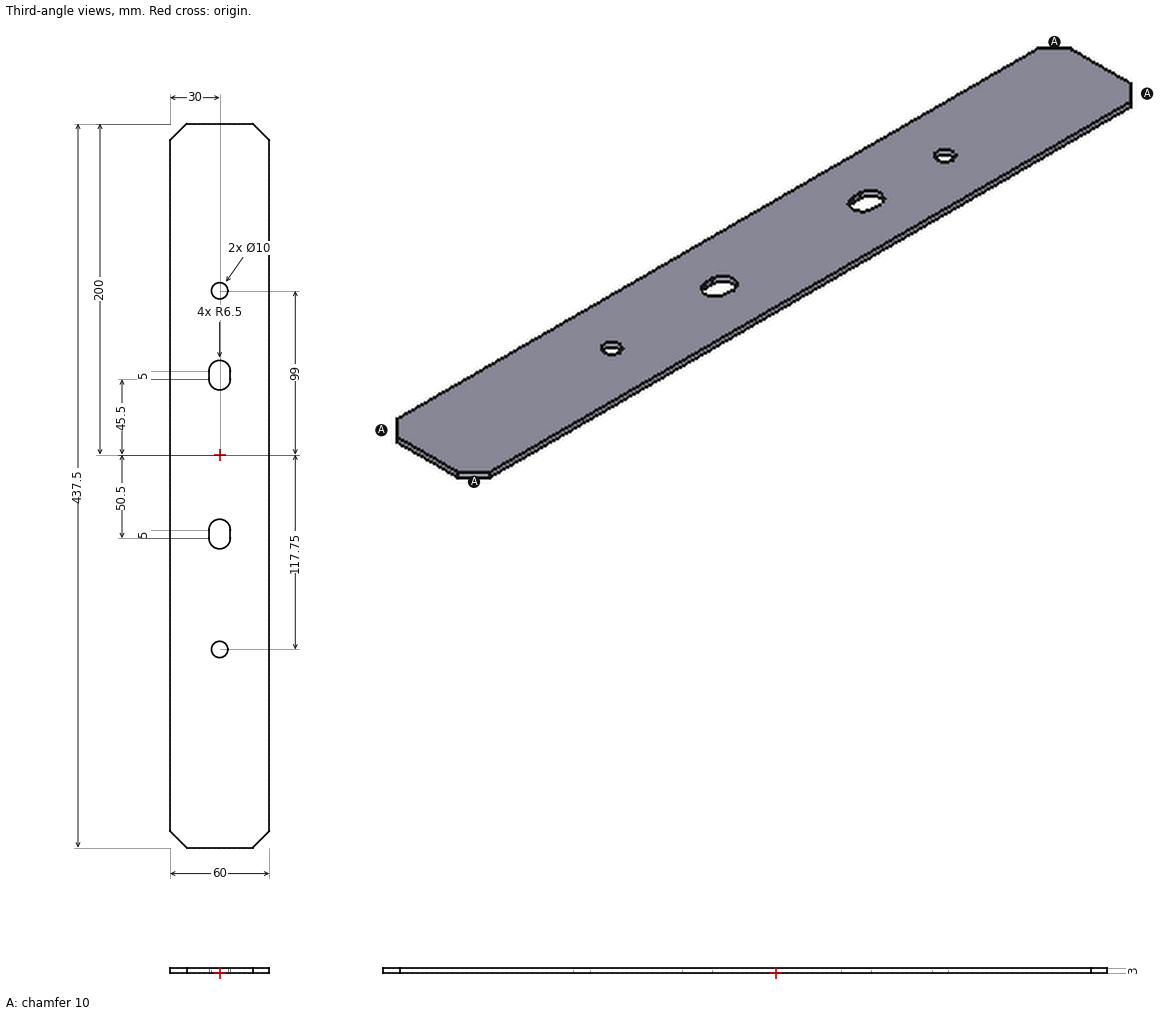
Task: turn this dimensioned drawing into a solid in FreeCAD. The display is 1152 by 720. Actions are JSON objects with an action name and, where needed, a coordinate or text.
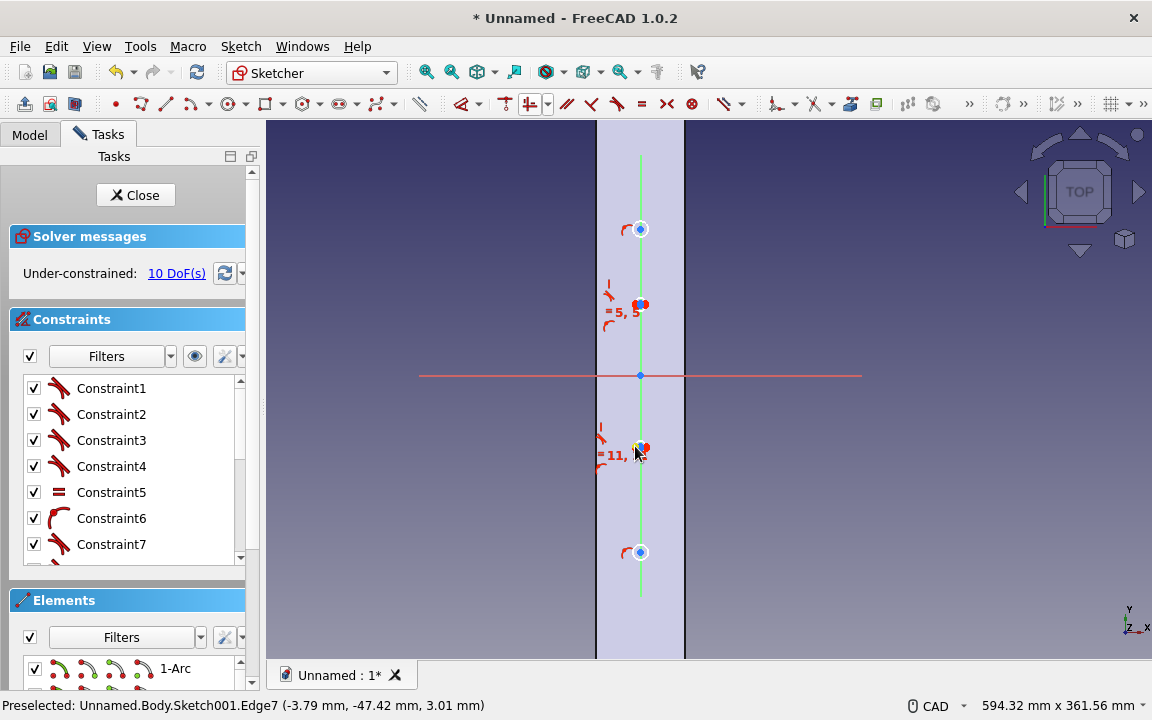
{"action": "scroll", "coordinate": [637, 310], "scroll_direction": "up", "scroll_amount": 8}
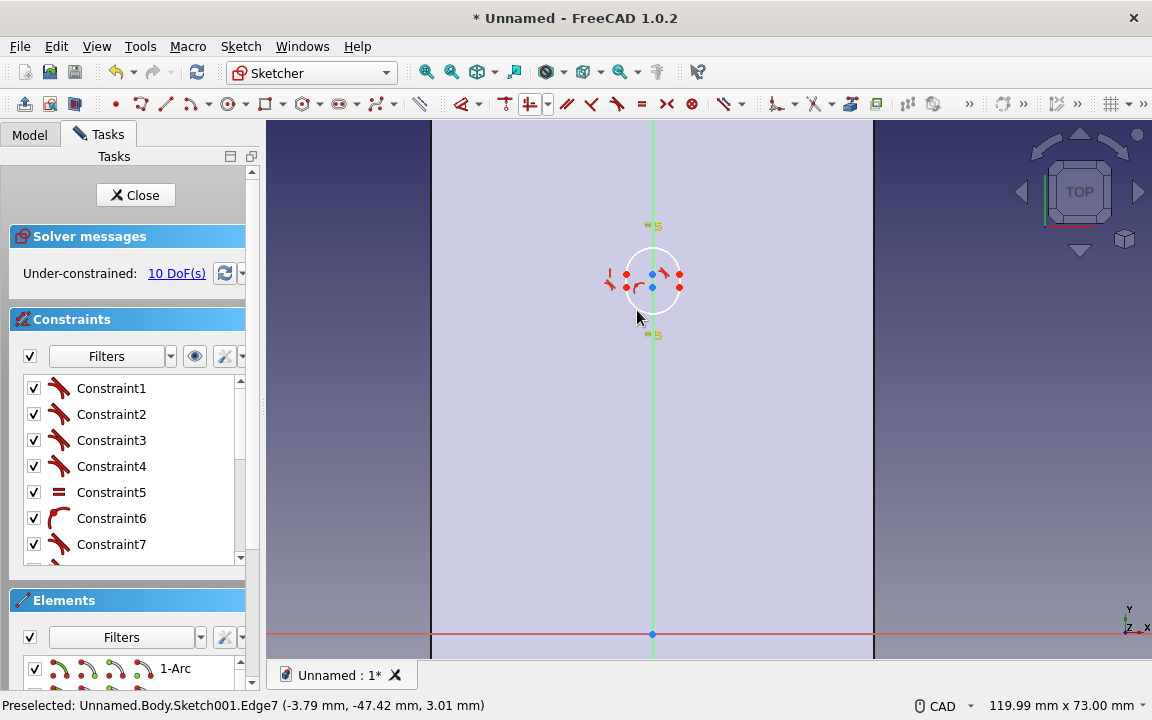
{"action": "left_click", "coordinate": [637, 309]}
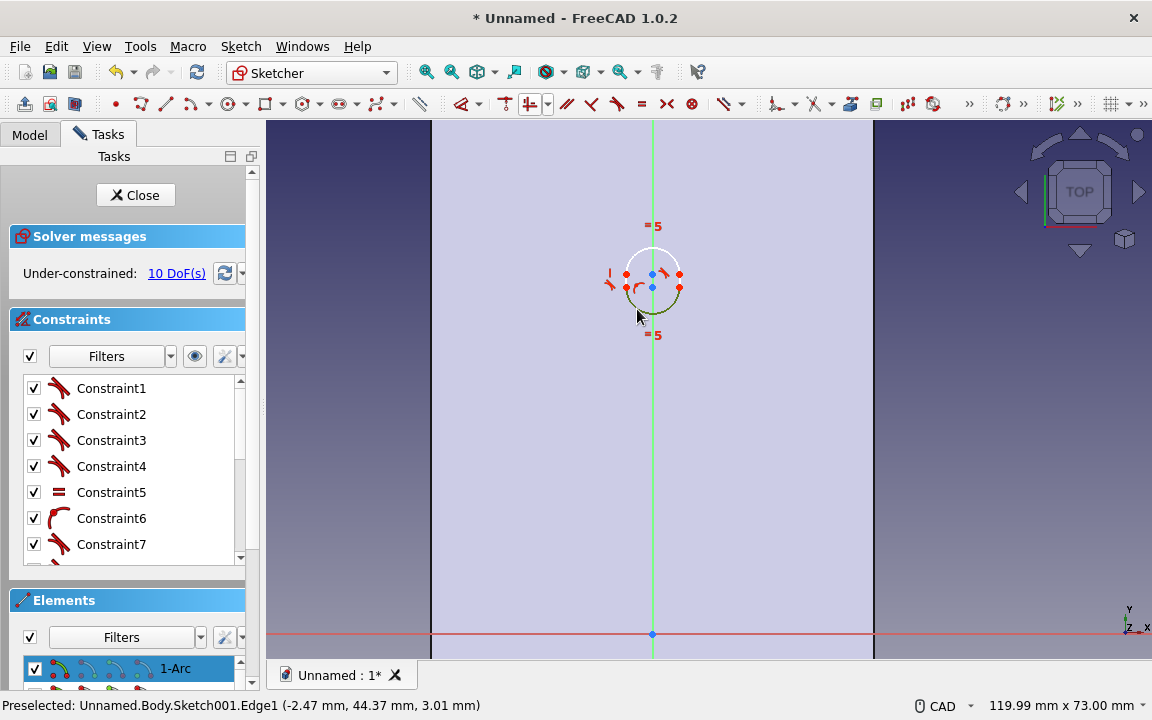
{"action": "scroll", "coordinate": [637, 310], "scroll_direction": "down", "scroll_amount": 8}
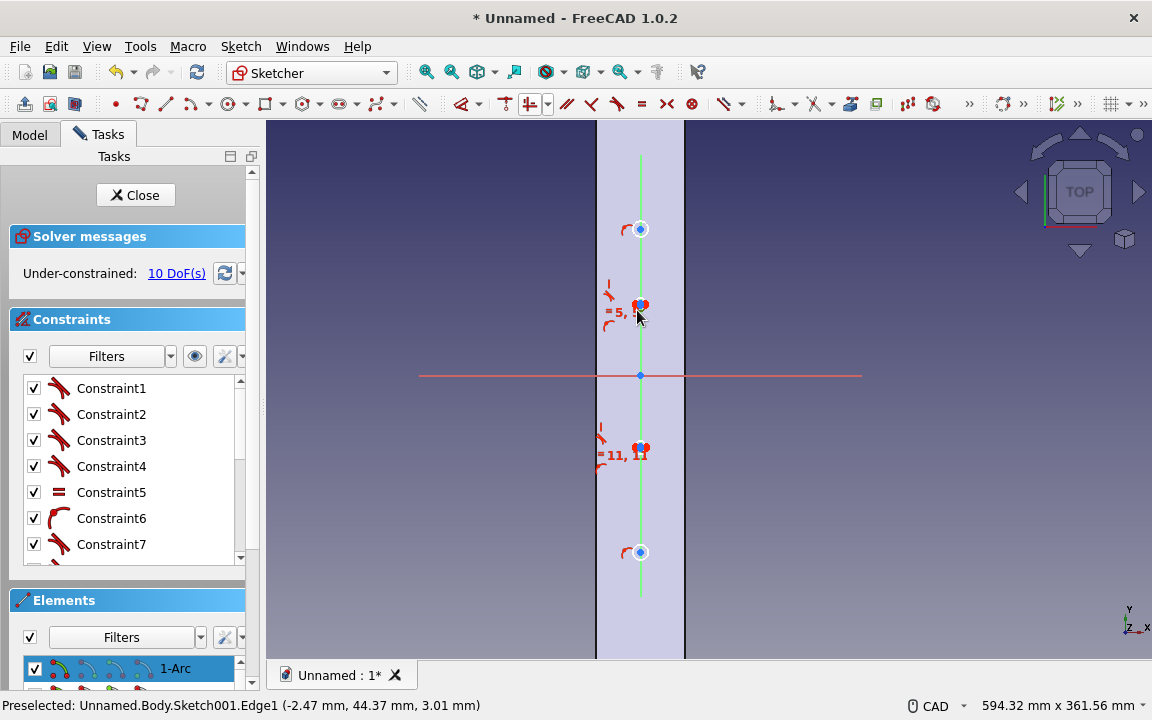
{"action": "scroll", "coordinate": [637, 453], "scroll_direction": "up", "scroll_amount": 8}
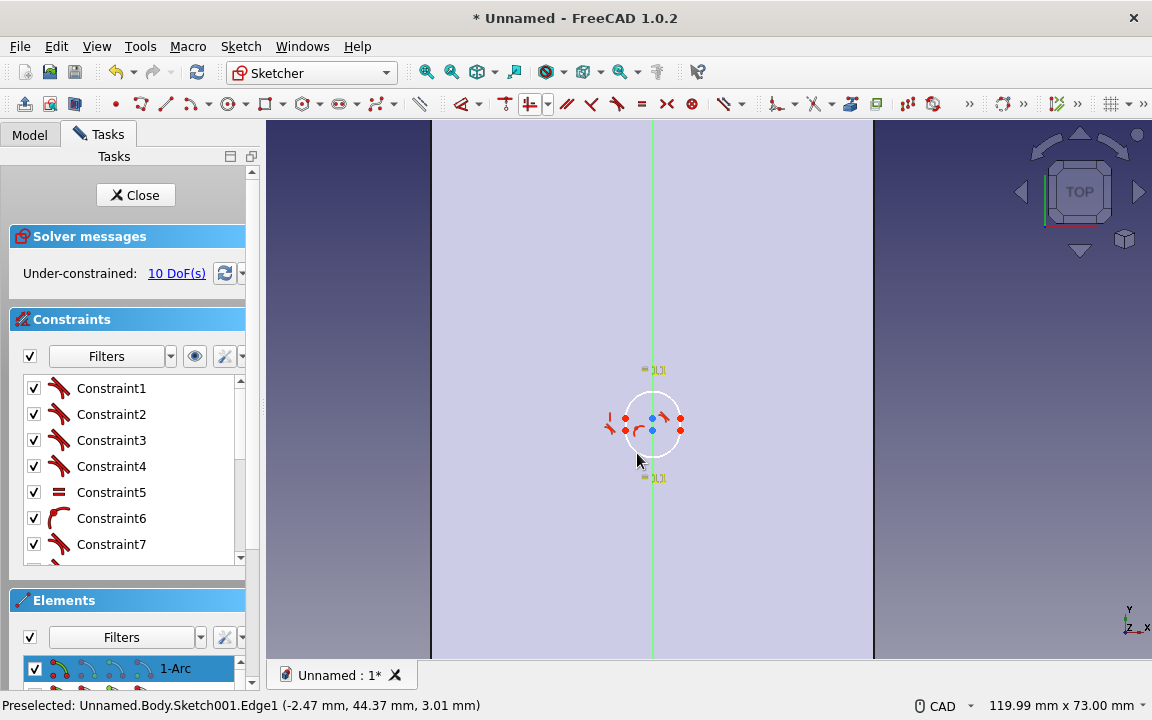
{"action": "left_click", "coordinate": [637, 452]}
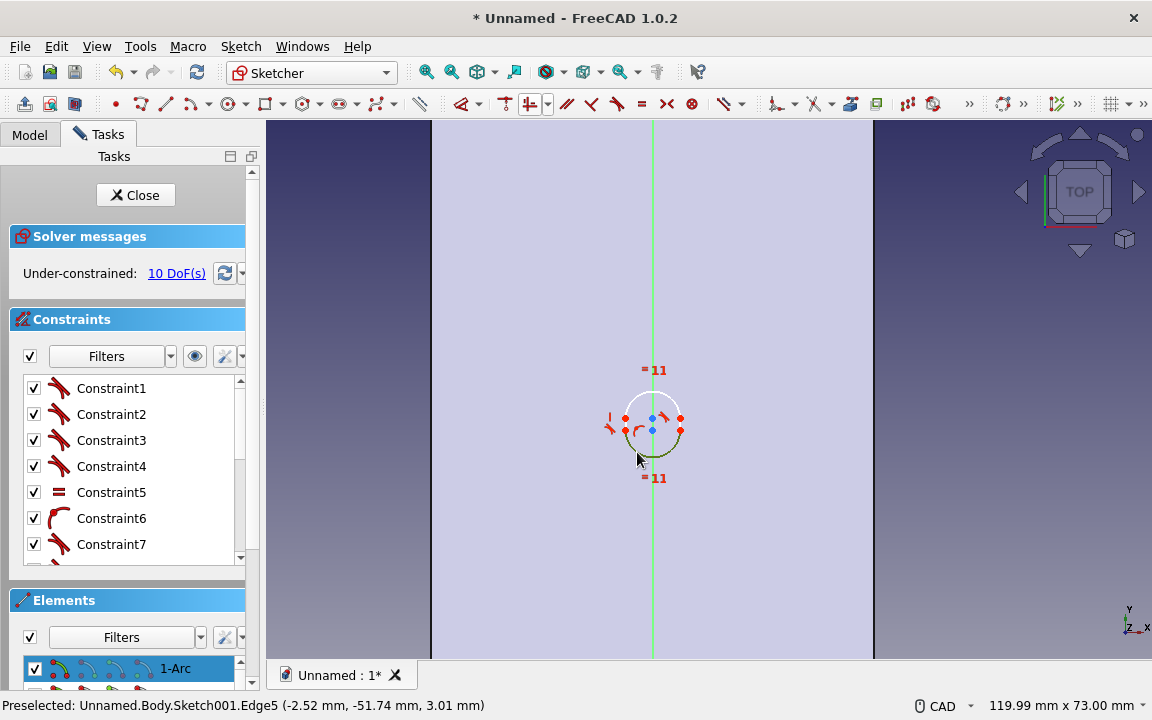
{"action": "left_click", "coordinate": [642, 104]}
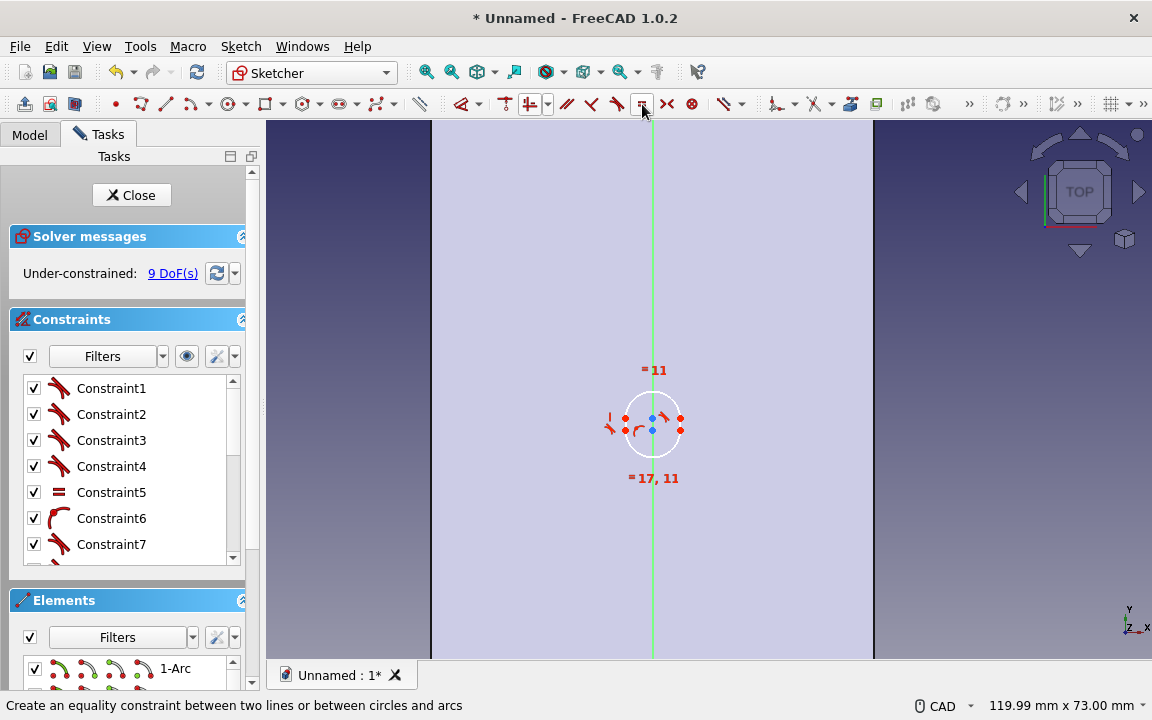
{"action": "scroll", "coordinate": [637, 453], "scroll_direction": "down", "scroll_amount": 8}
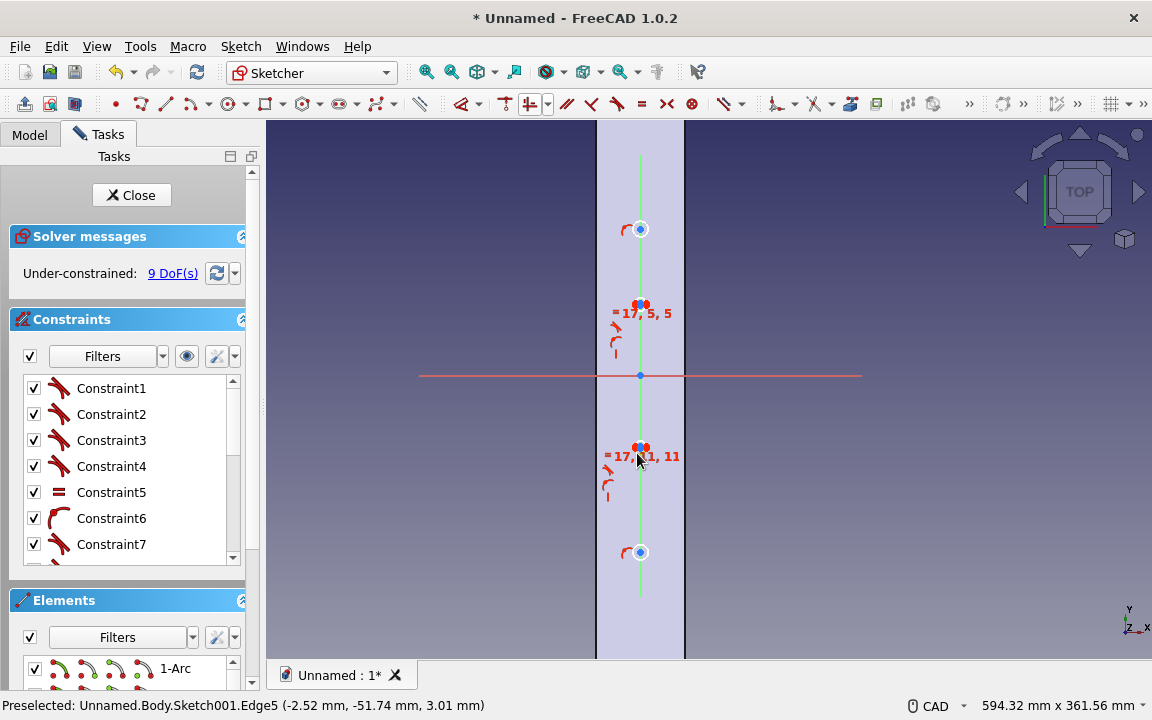
{"action": "scroll", "coordinate": [646, 224], "scroll_direction": "up", "scroll_amount": 5}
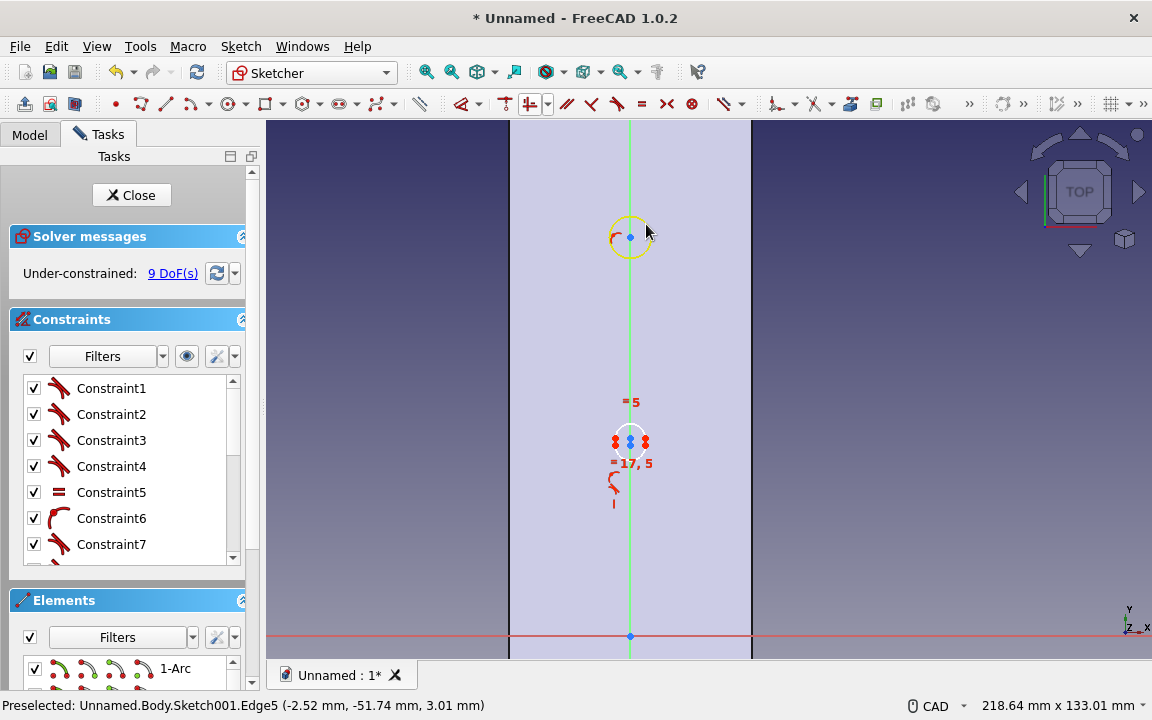
{"action": "left_click", "coordinate": [645, 223]}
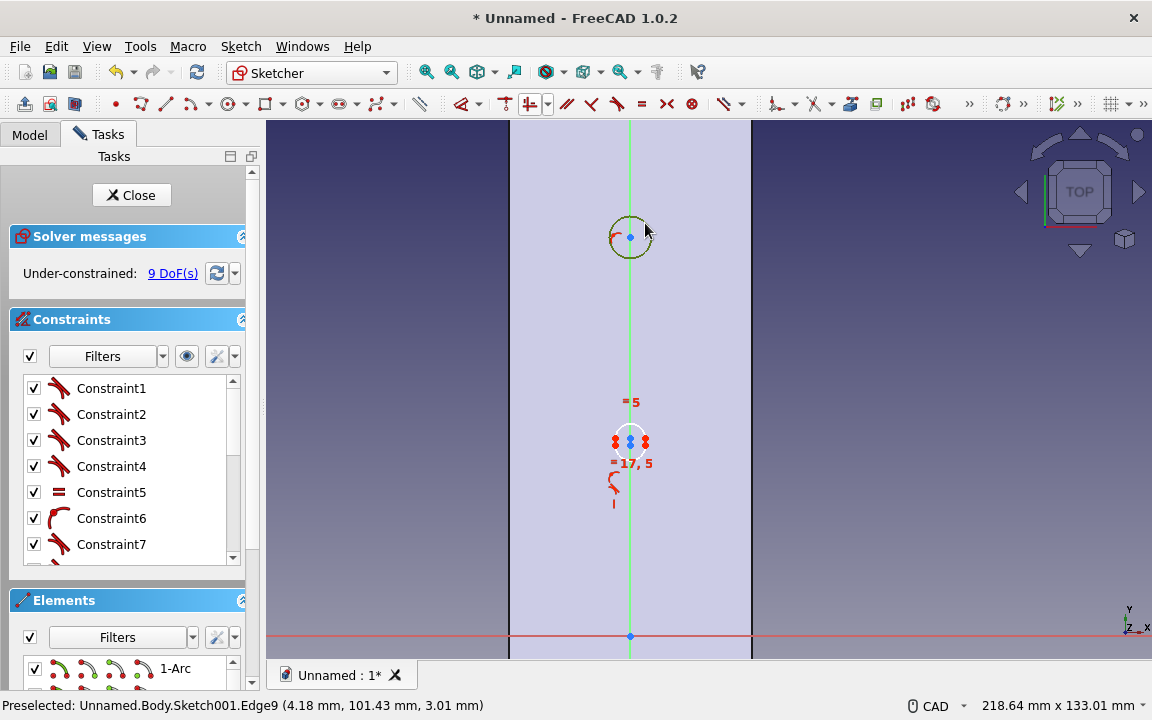
{"action": "scroll", "coordinate": [646, 224], "scroll_direction": "down", "scroll_amount": 5}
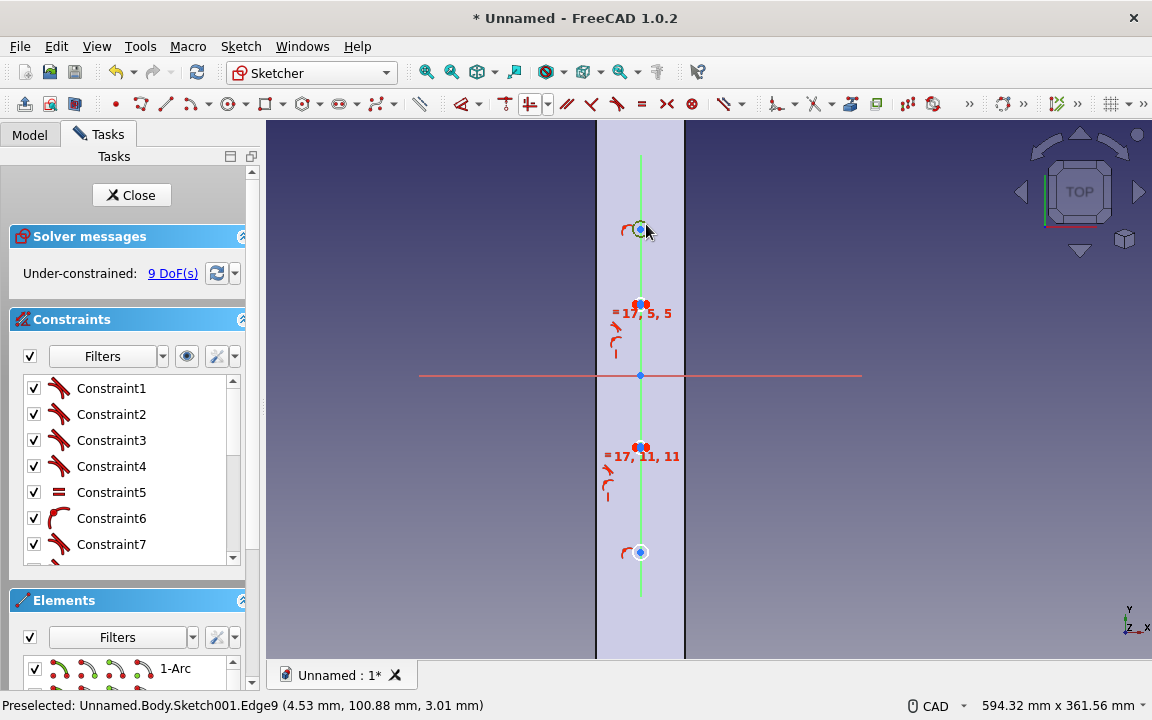
{"action": "scroll", "coordinate": [646, 547], "scroll_direction": "up", "scroll_amount": 5}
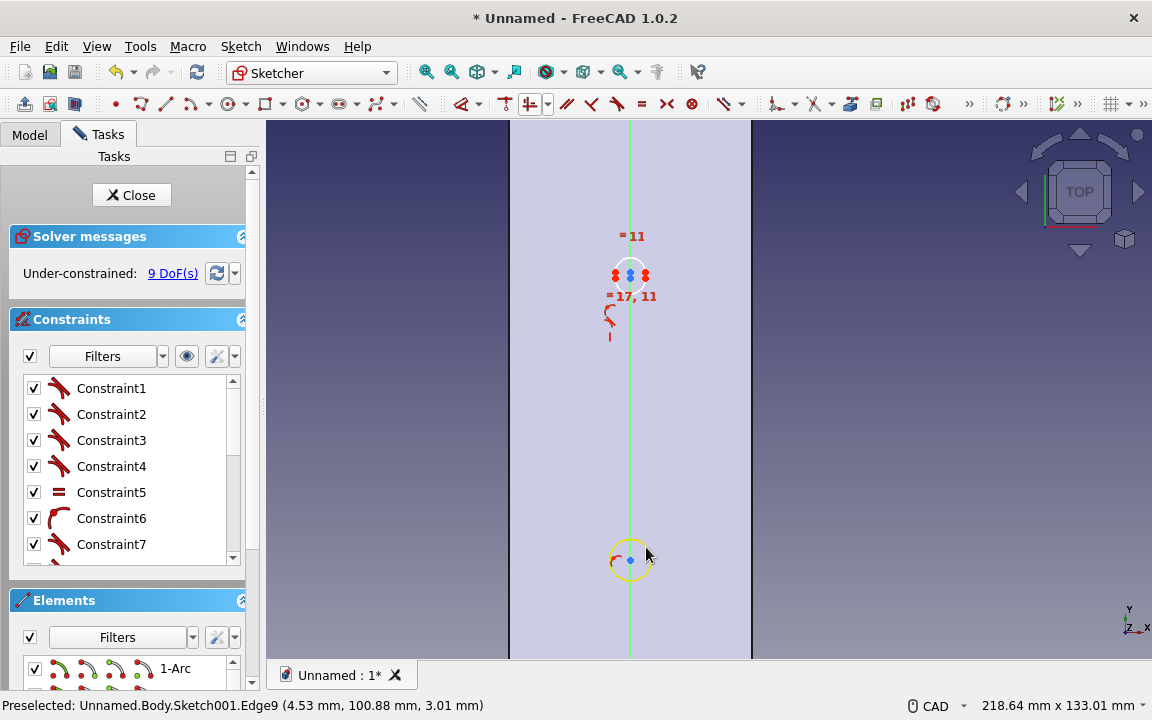
{"action": "left_click", "coordinate": [645, 545]}